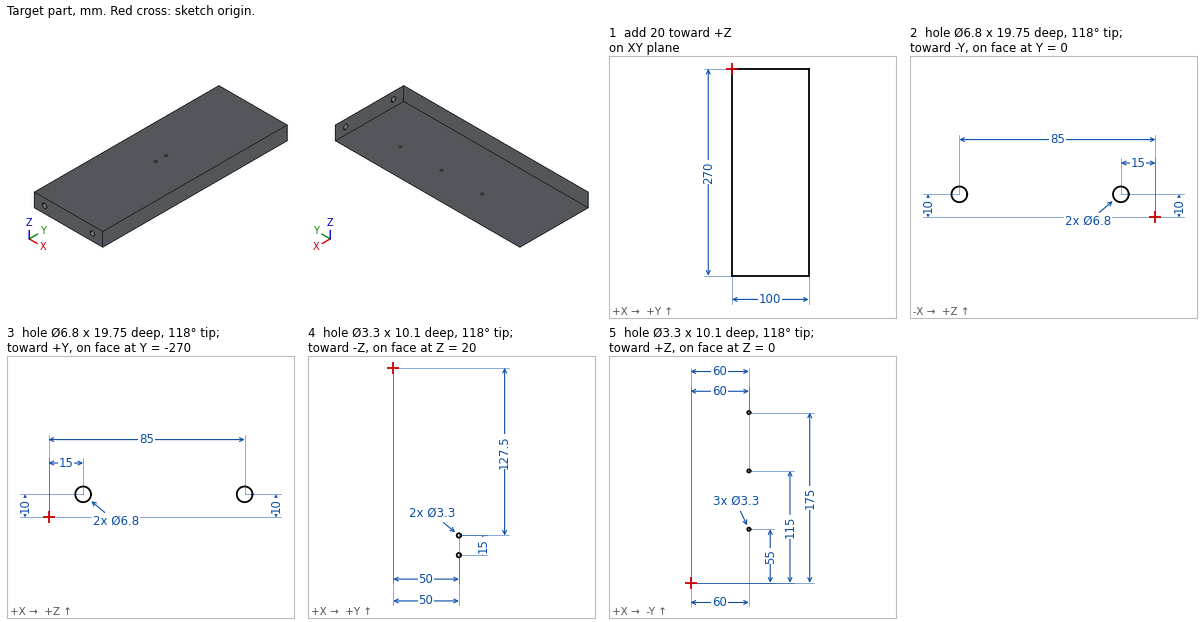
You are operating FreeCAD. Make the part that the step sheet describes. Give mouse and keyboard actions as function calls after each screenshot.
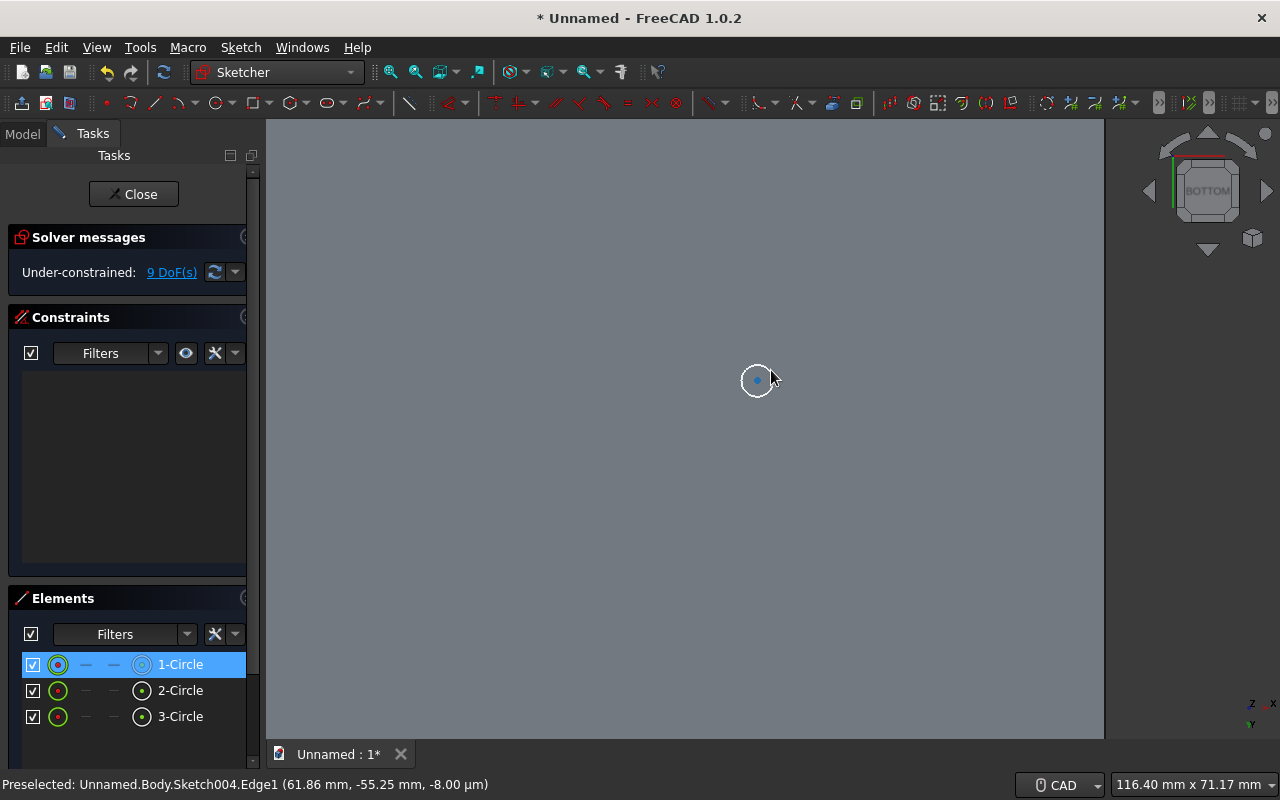
click(768, 370)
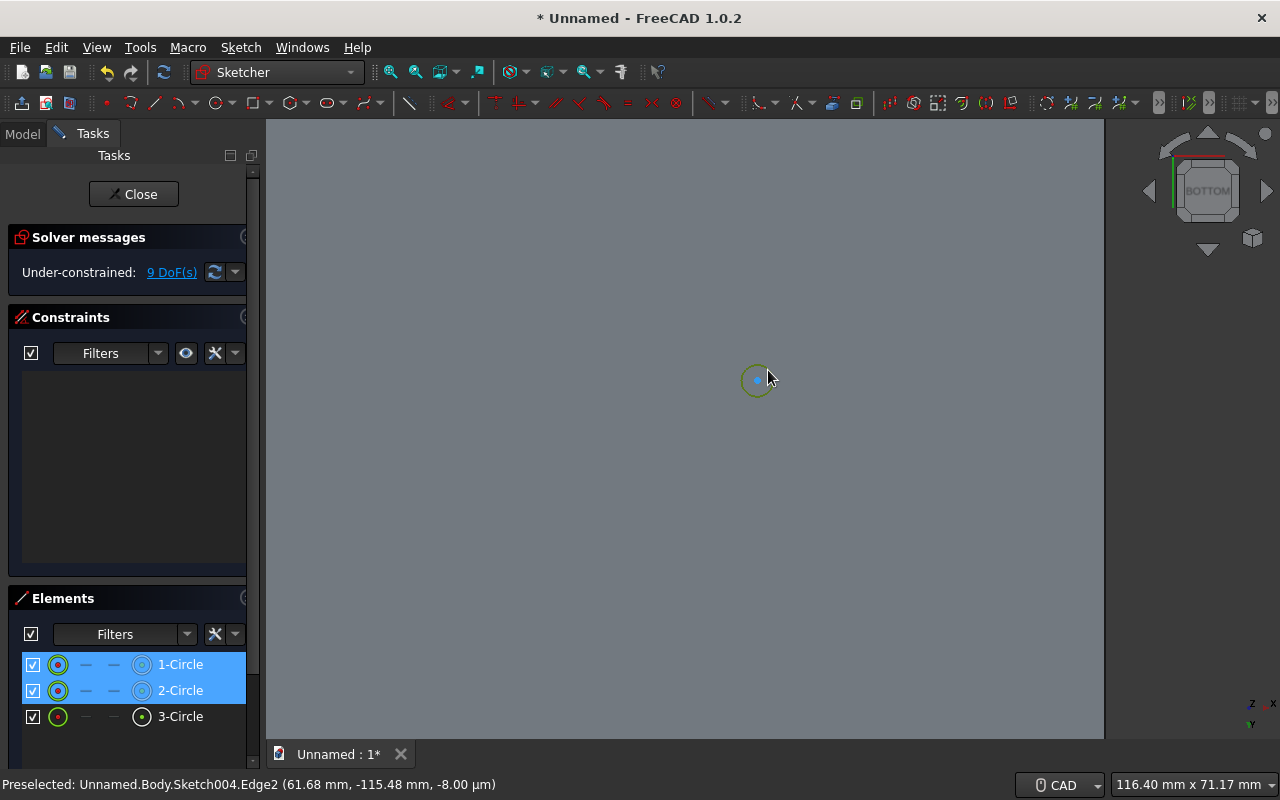
scroll(771, 370, down, 7)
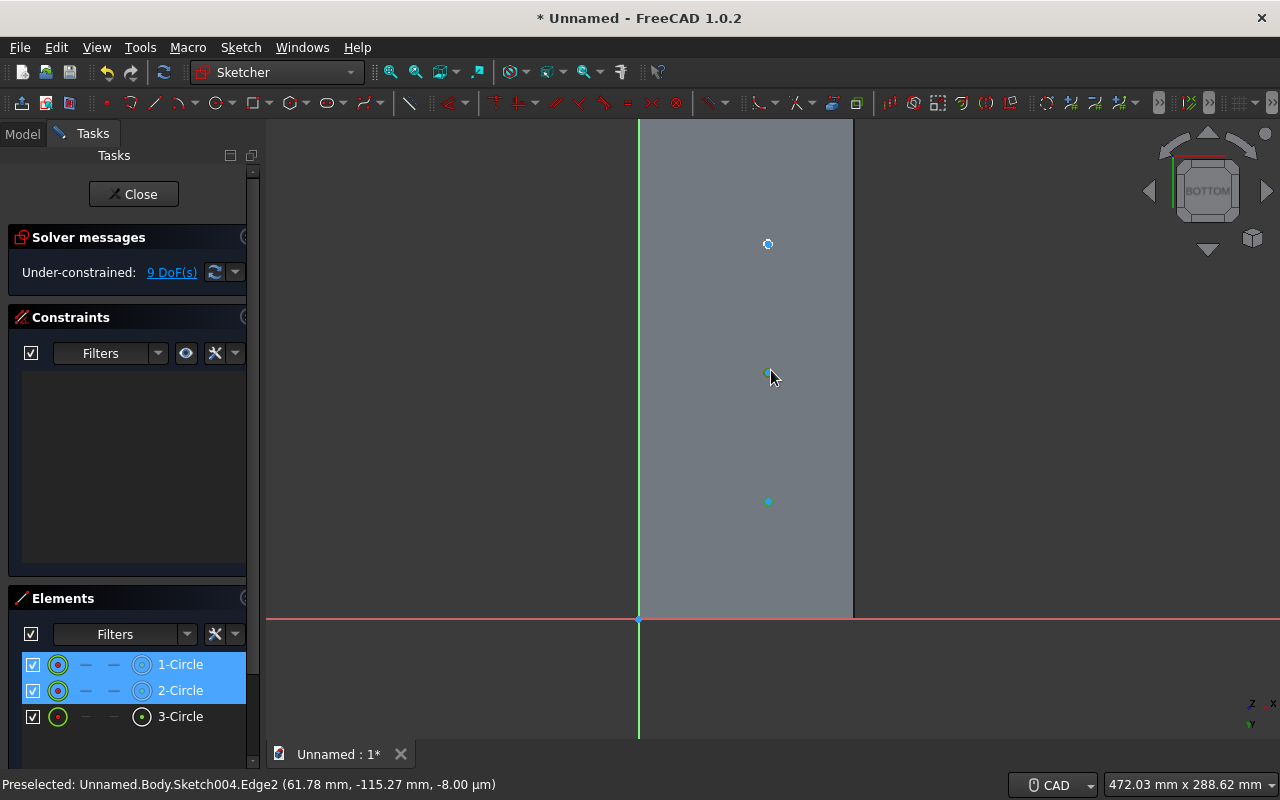
scroll(771, 241, up, 7)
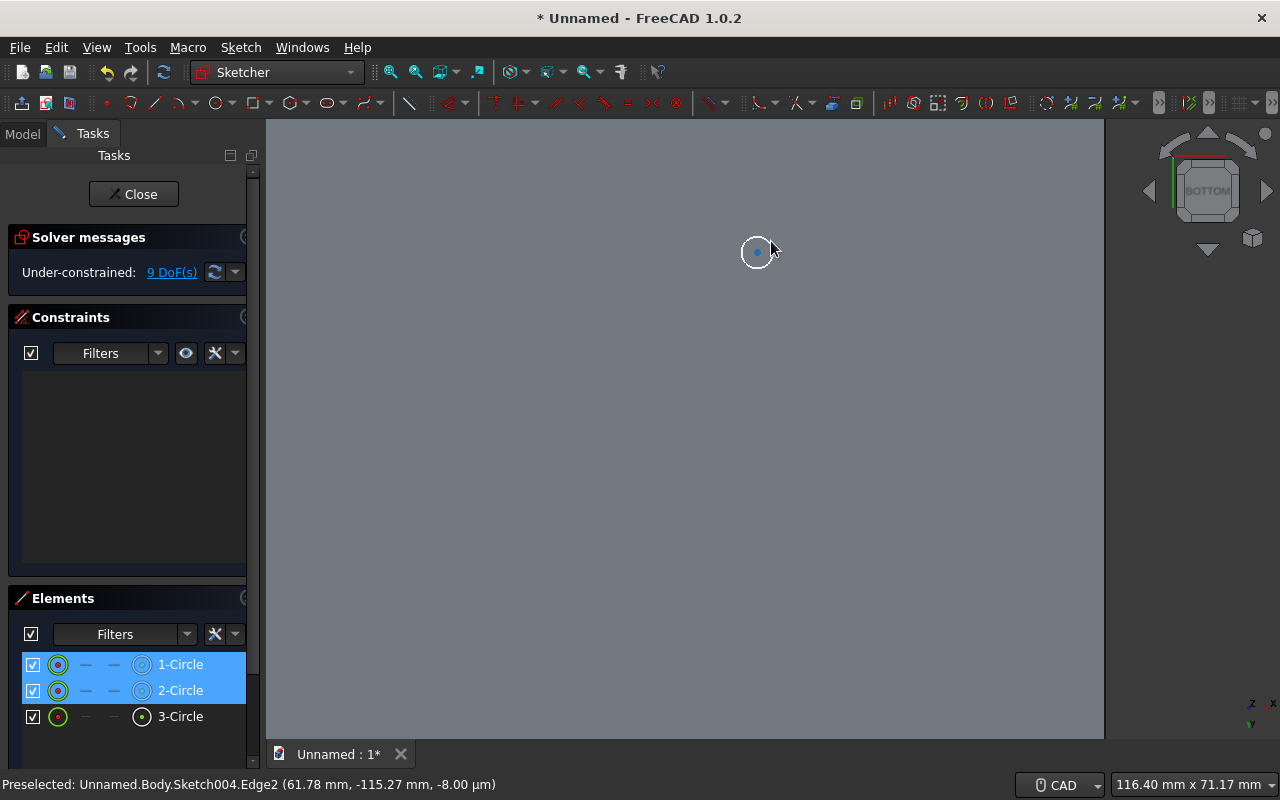
click(768, 241)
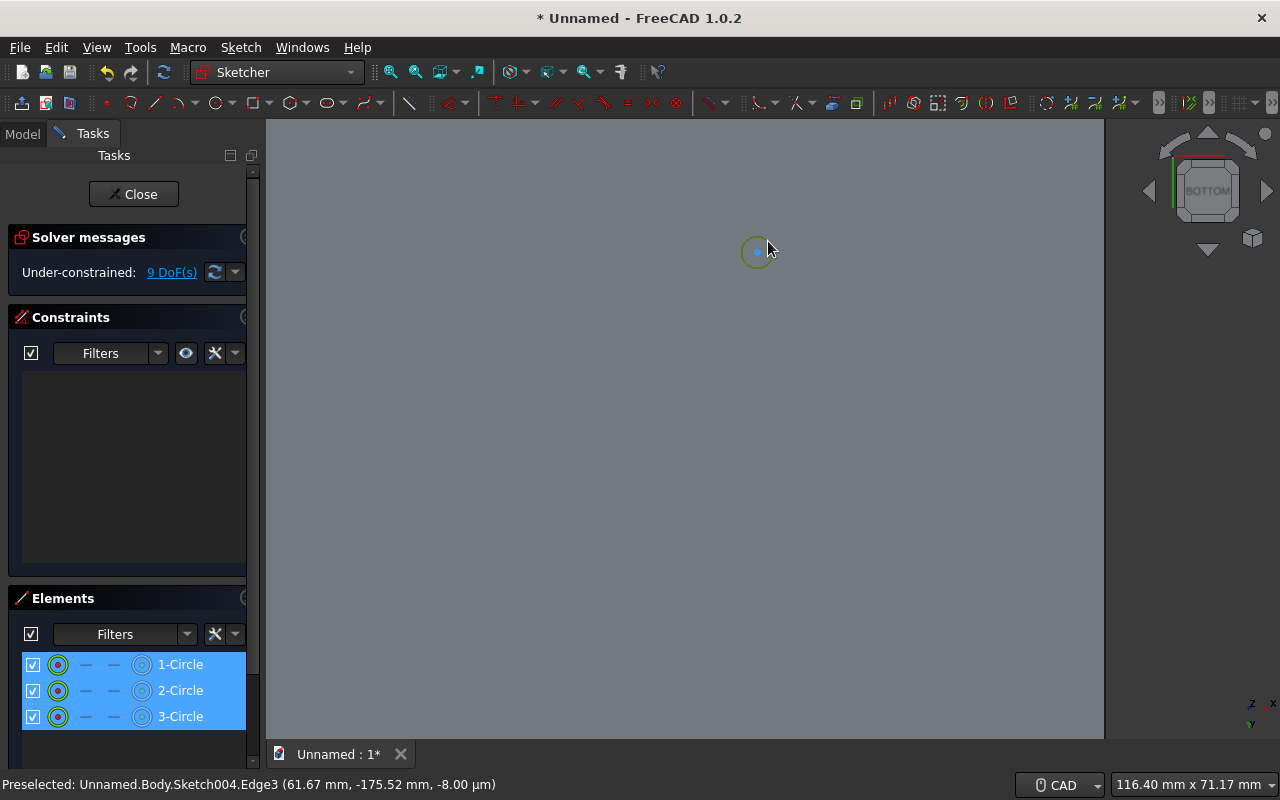
key(e)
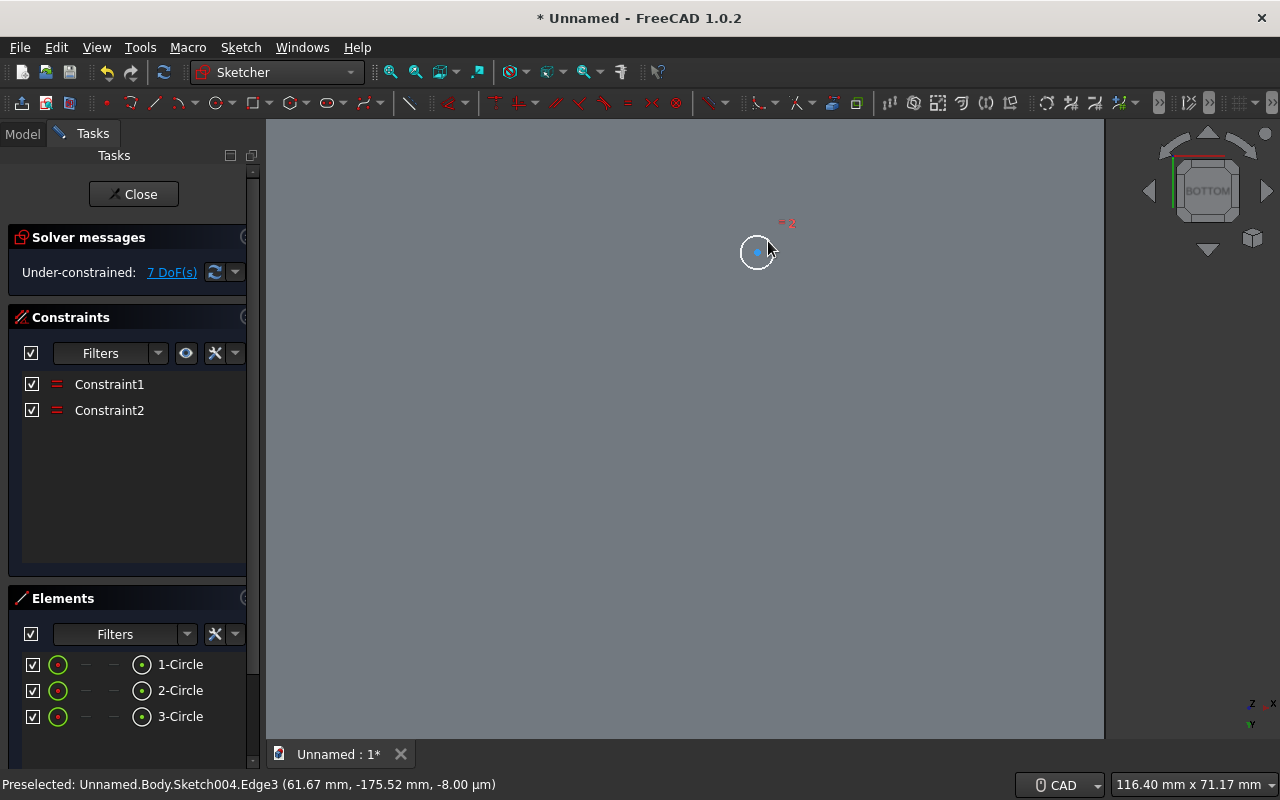
key(d)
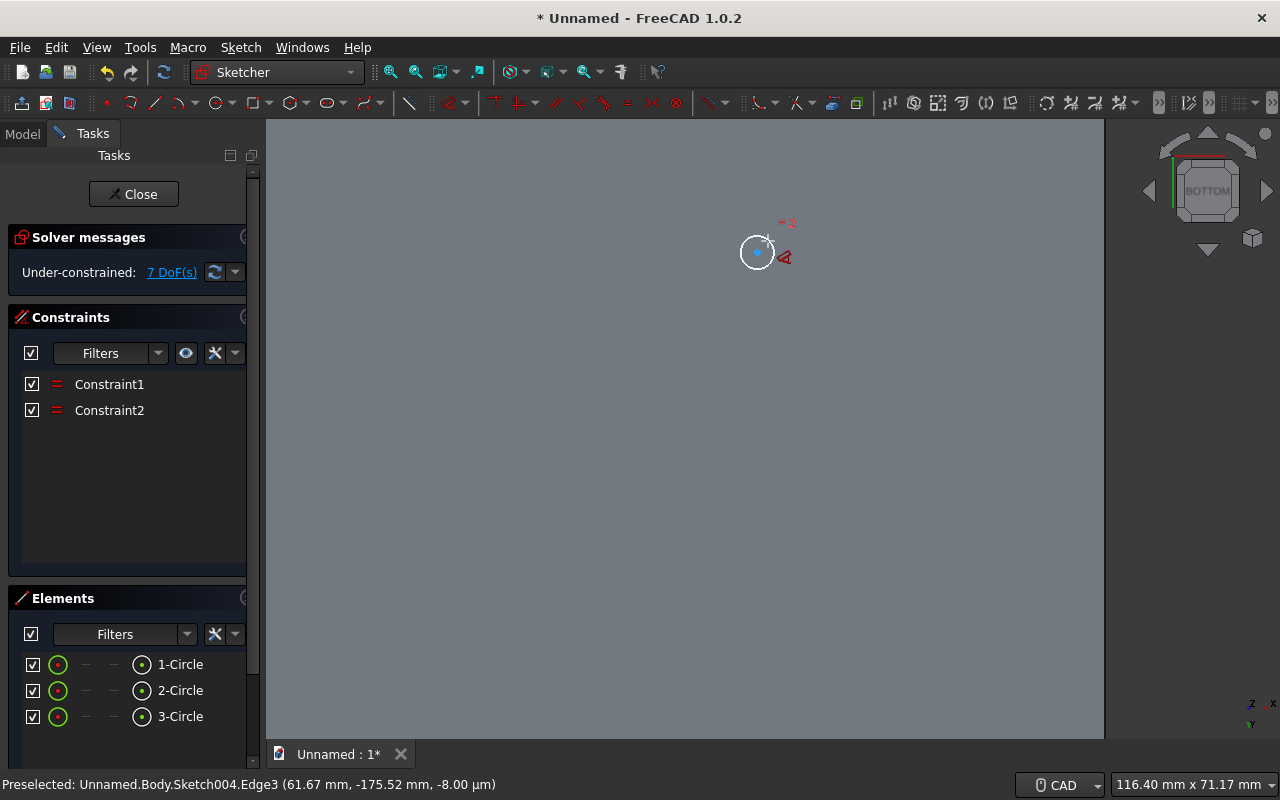
scroll(771, 241, down, 7)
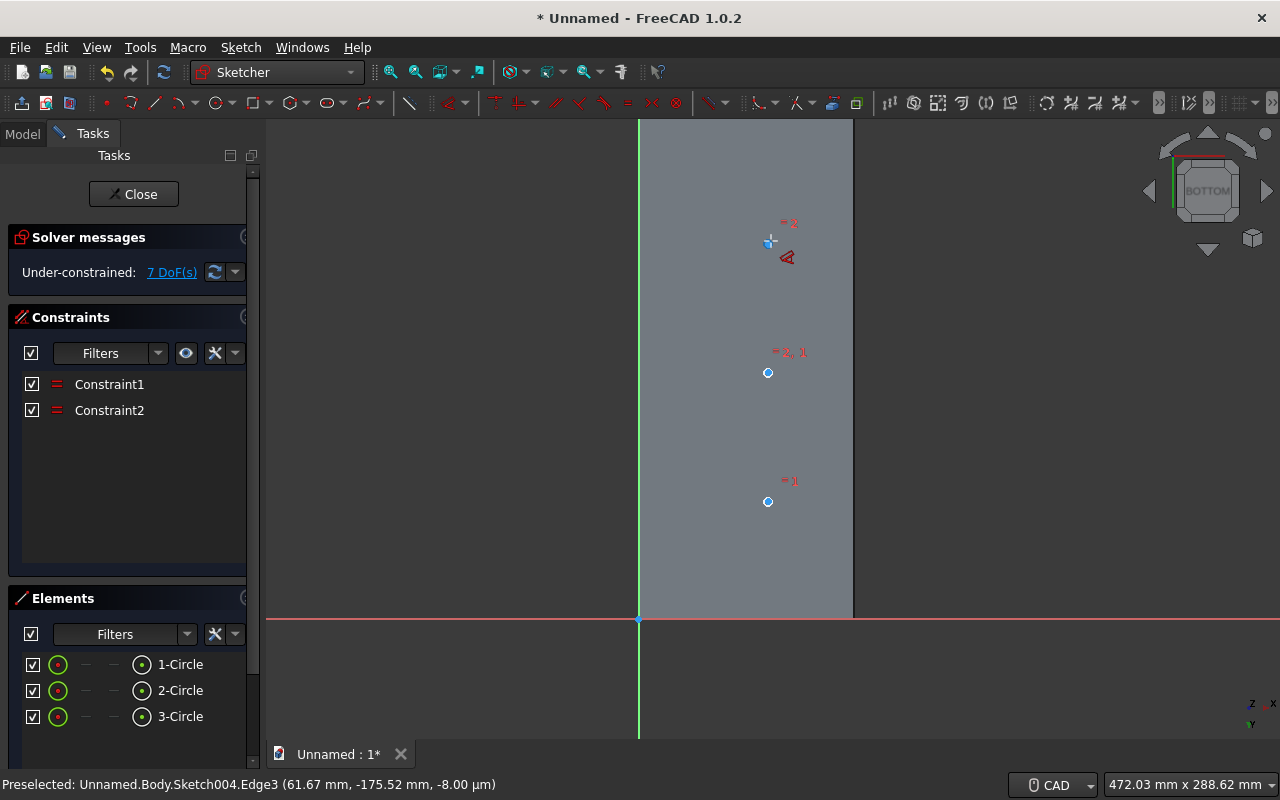
scroll(771, 499, up, 9)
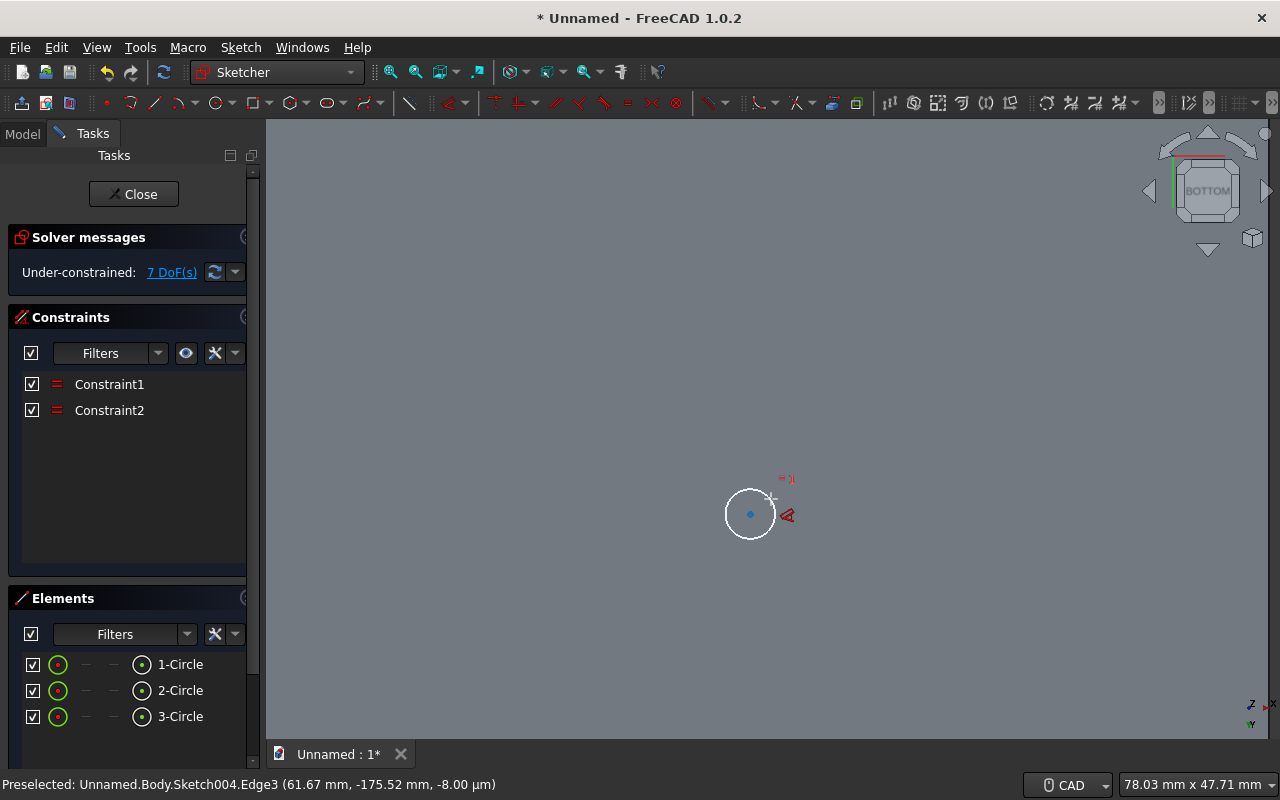
click(768, 496)
click(790, 473)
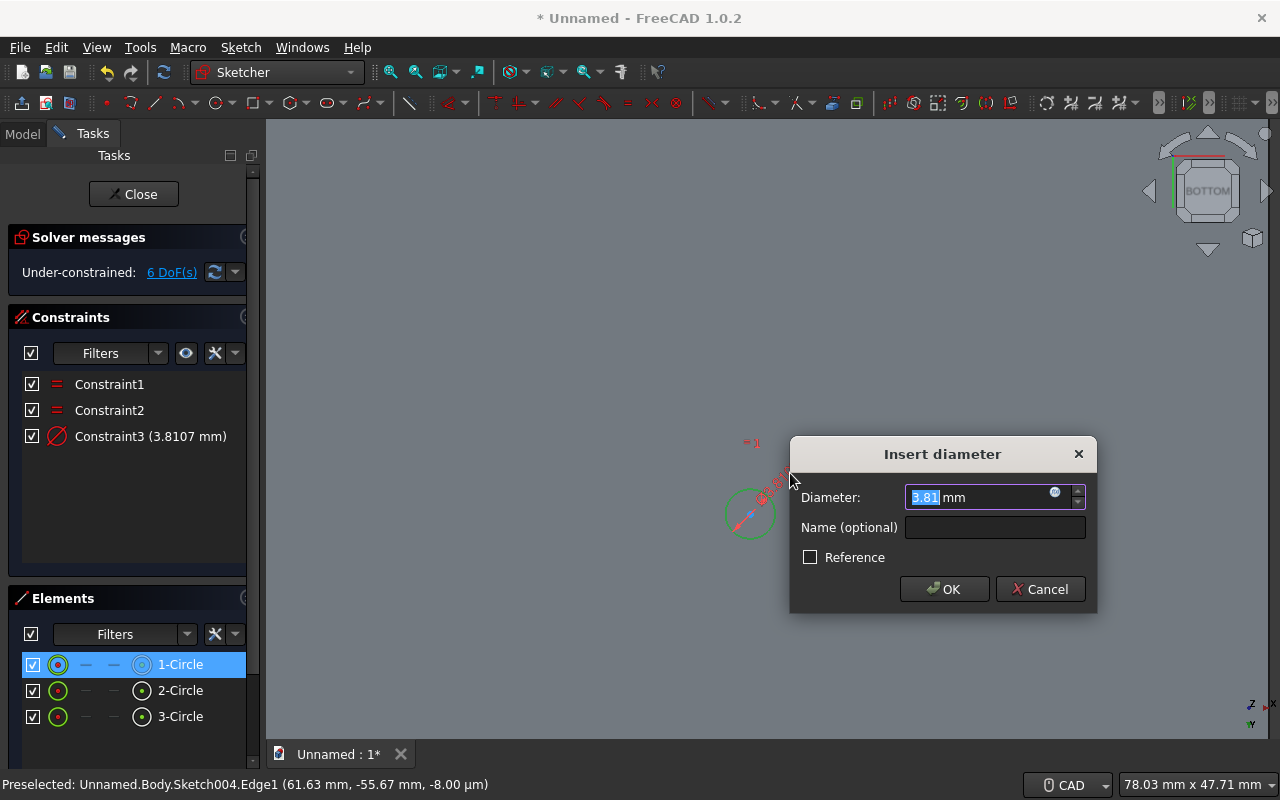
text(3.3)
key(Return)